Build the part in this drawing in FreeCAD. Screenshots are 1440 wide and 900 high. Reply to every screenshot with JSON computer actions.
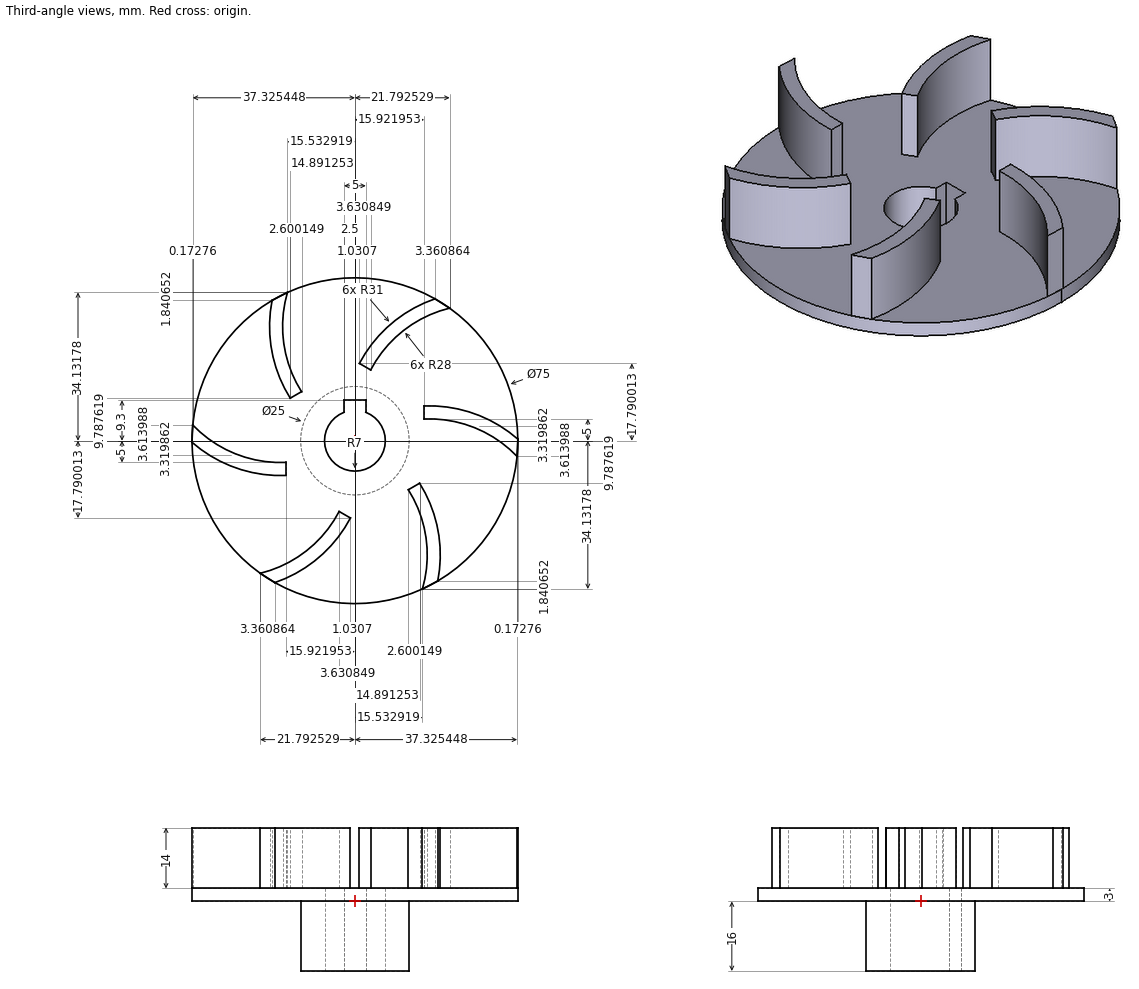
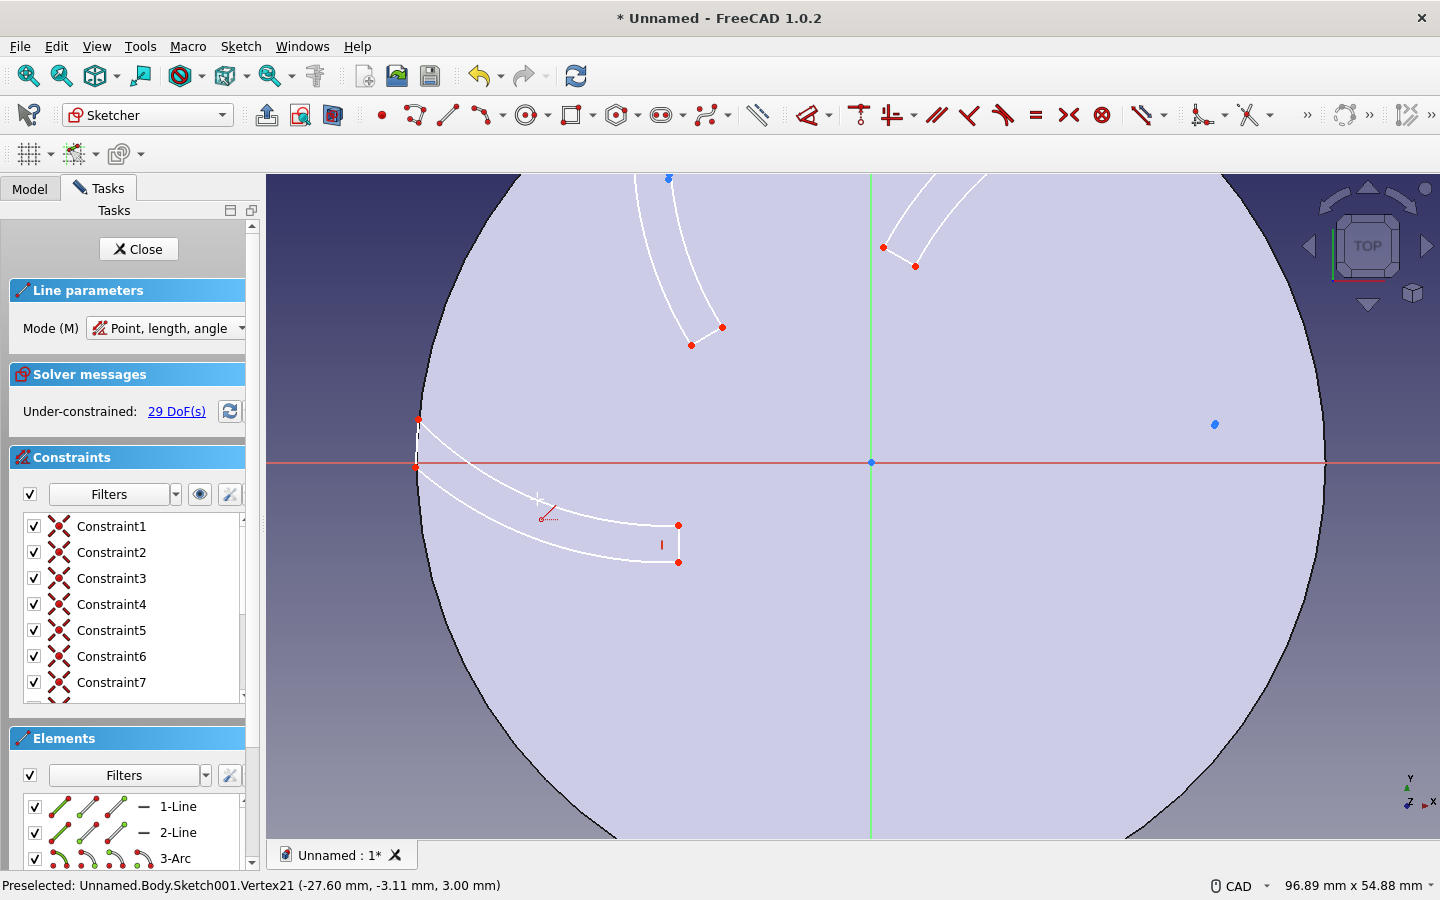
{"action": "scroll", "coordinate": [679, 560], "scroll_direction": "down", "scroll_amount": 3}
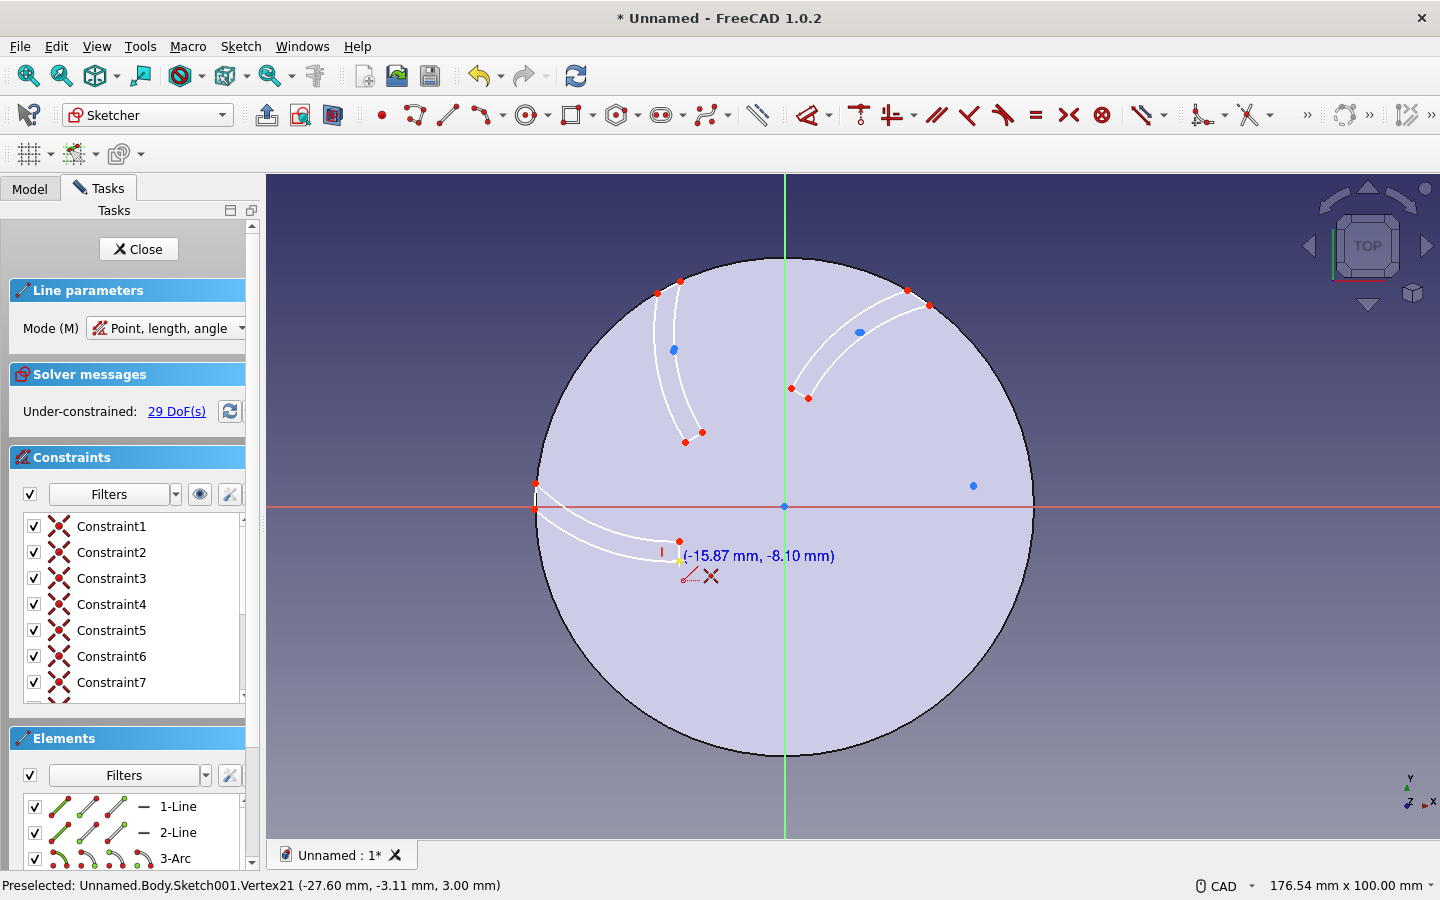
{"action": "left_click", "coordinate": [640, 710]}
{"action": "left_click", "coordinate": [662, 724]}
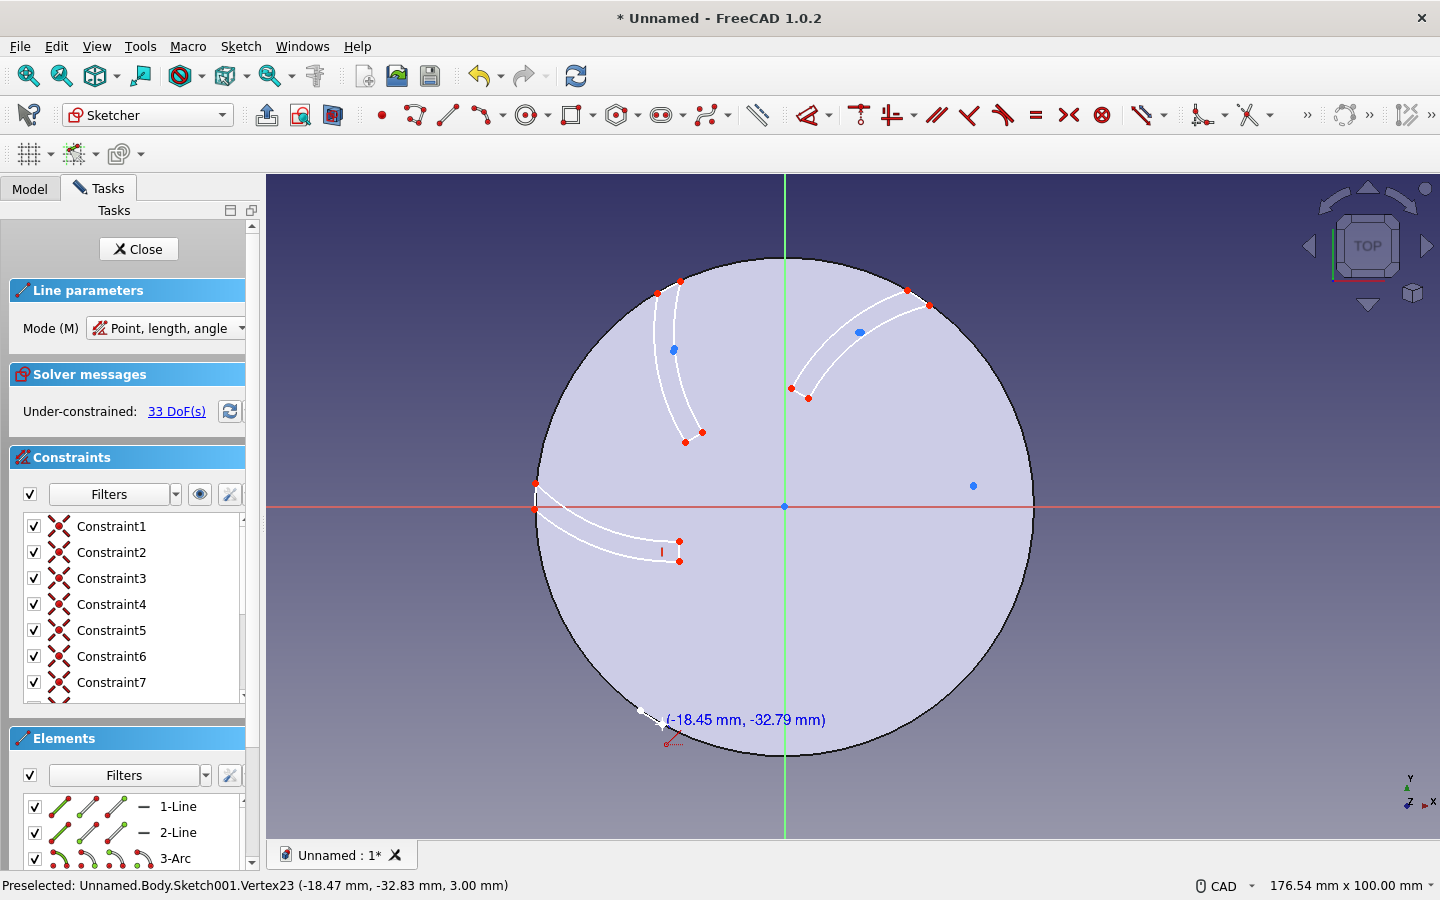
{"action": "scroll", "coordinate": [778, 625], "scroll_direction": "up", "scroll_amount": 5}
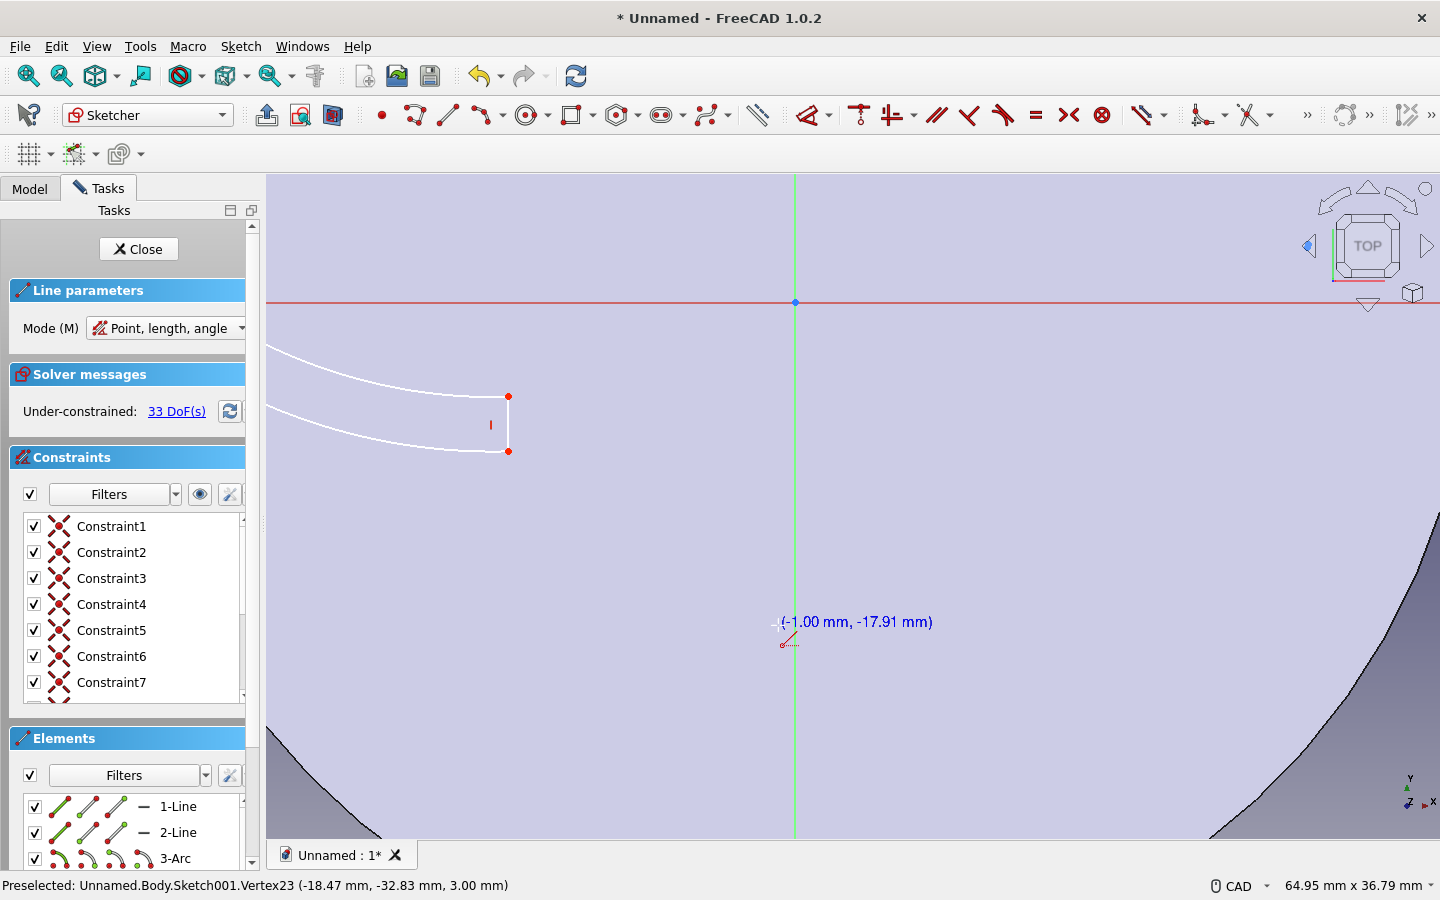
{"action": "left_click", "coordinate": [777, 624]}
{"action": "left_click", "coordinate": [730, 597]}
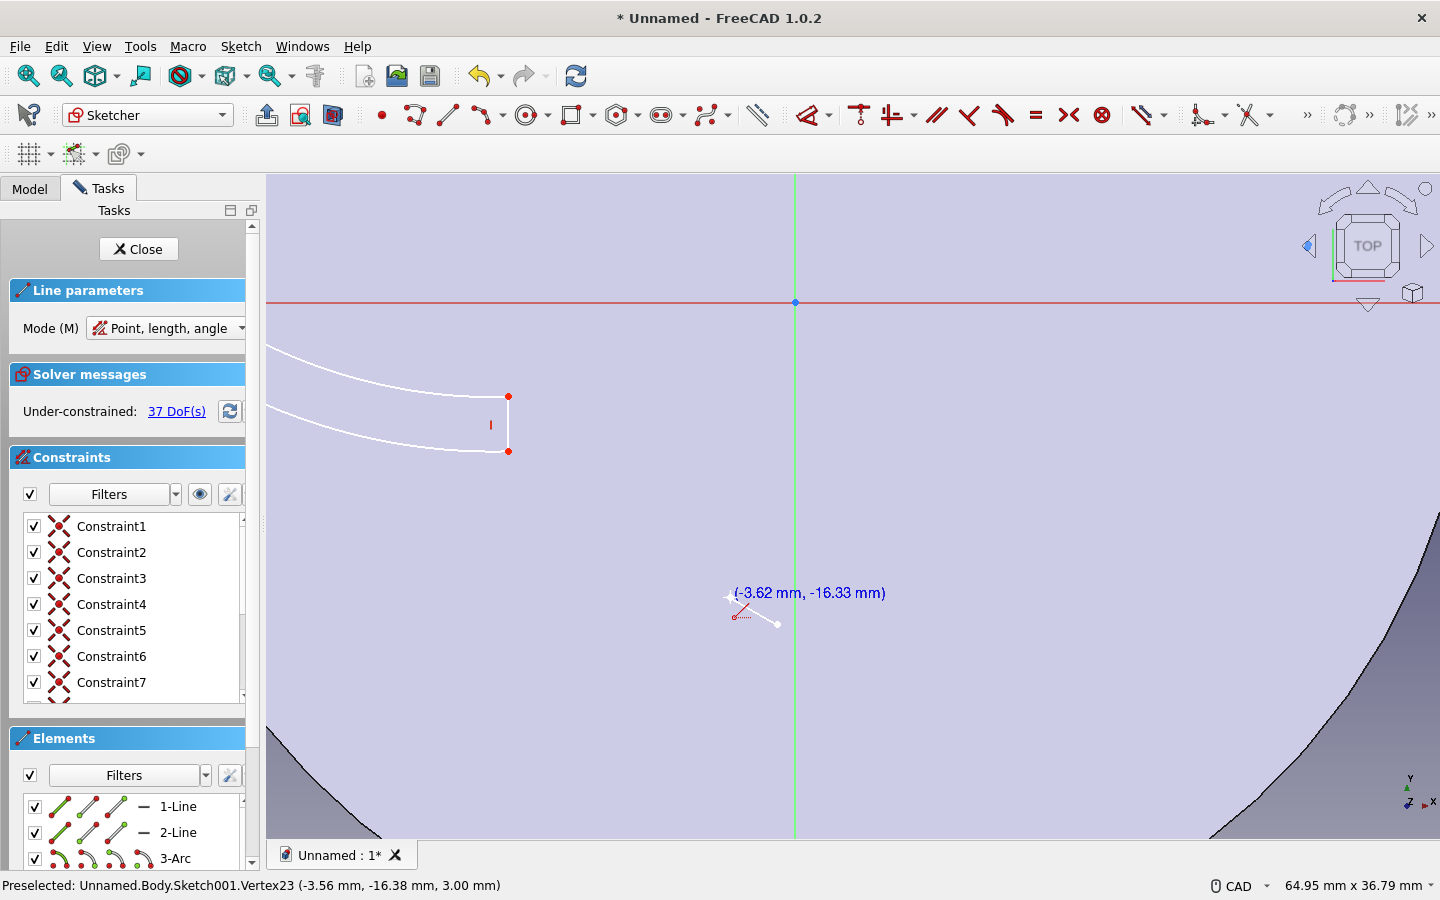
{"action": "key", "text": "g 3 a"}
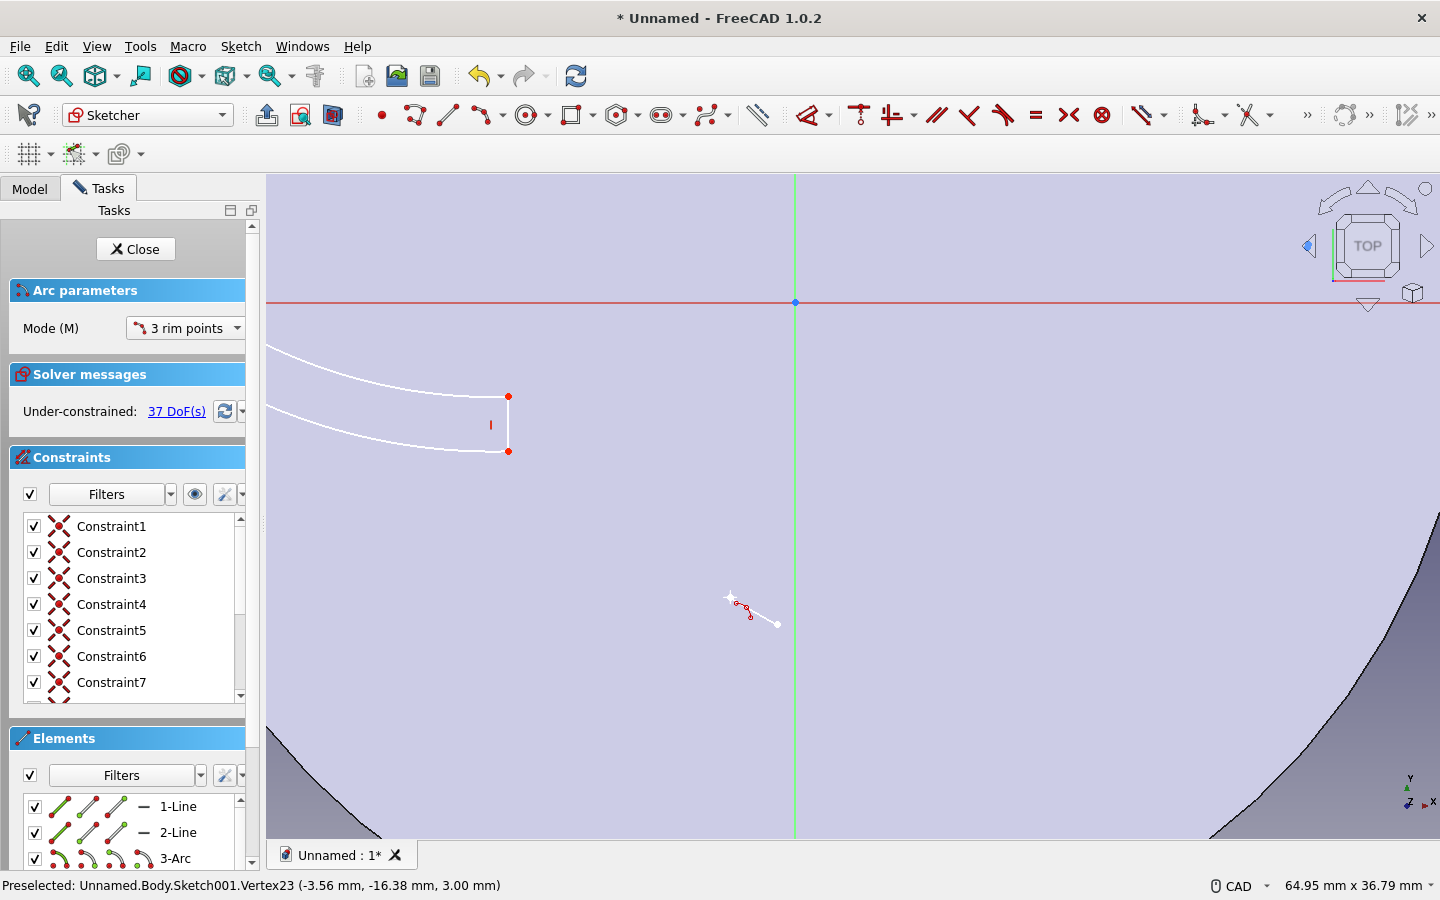
{"action": "scroll", "coordinate": [778, 625], "scroll_direction": "down", "scroll_amount": 5}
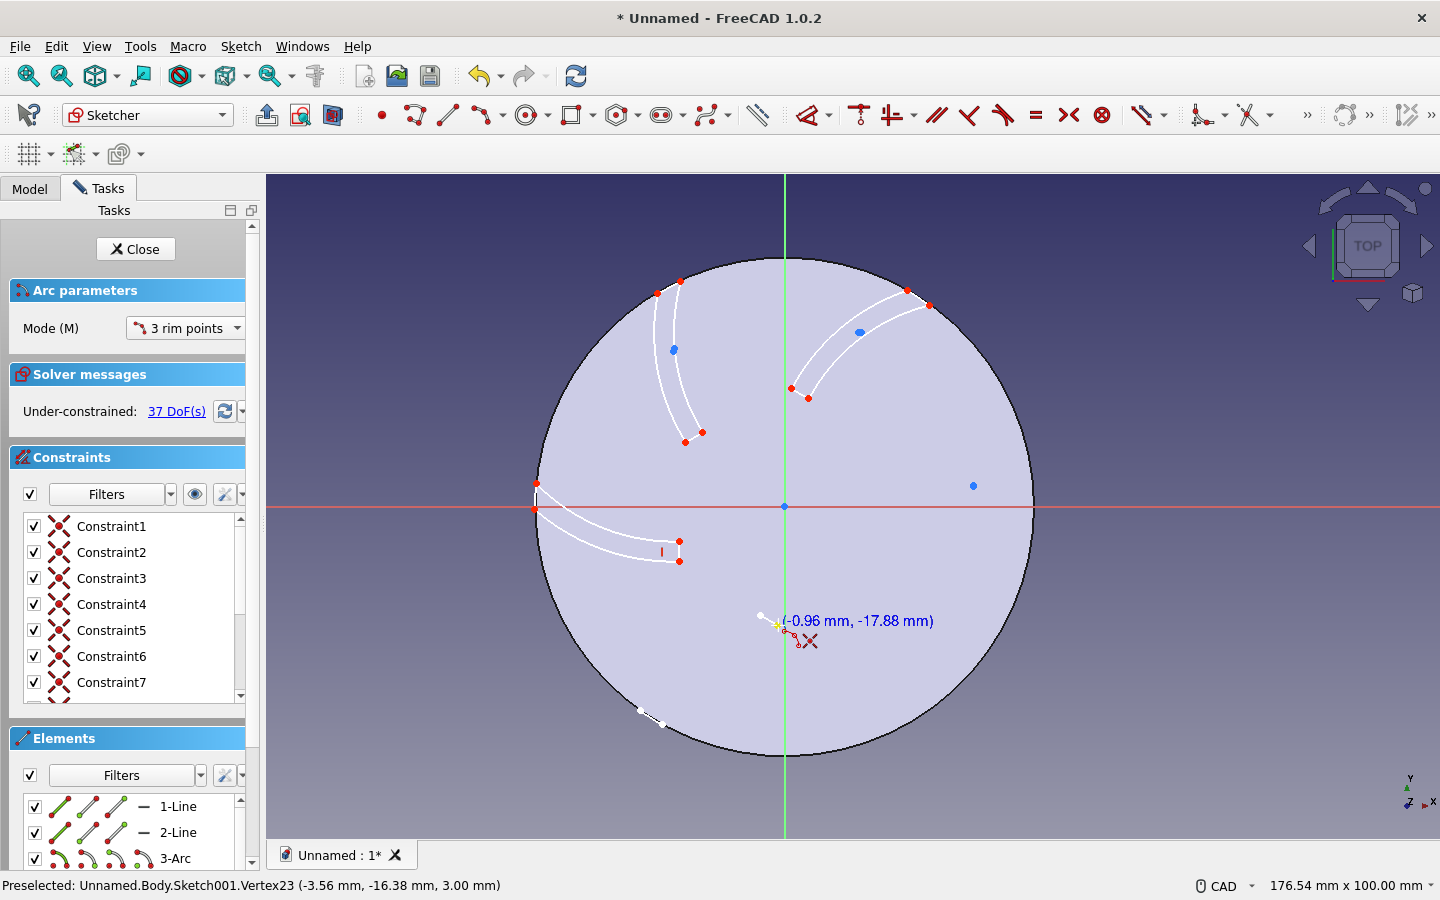
{"action": "left_click", "coordinate": [662, 725]}